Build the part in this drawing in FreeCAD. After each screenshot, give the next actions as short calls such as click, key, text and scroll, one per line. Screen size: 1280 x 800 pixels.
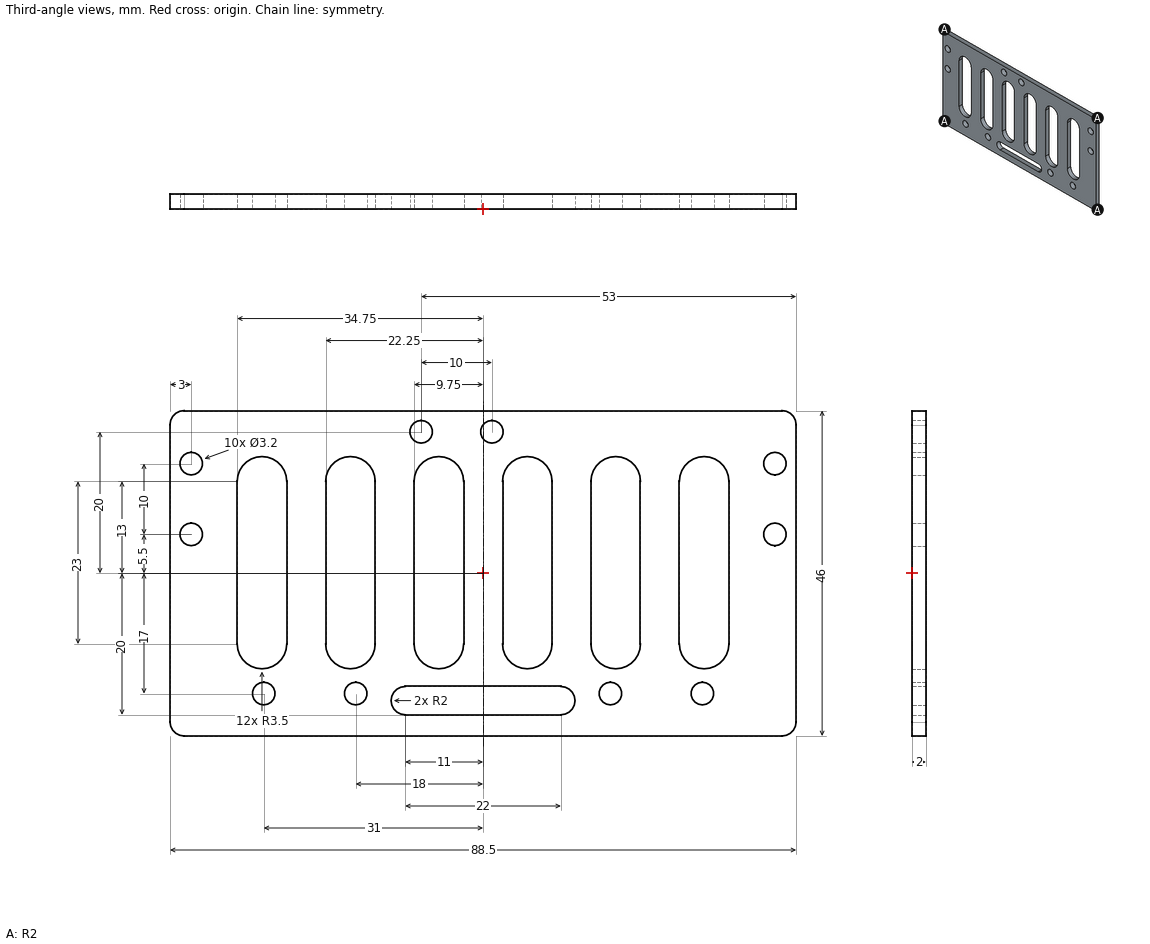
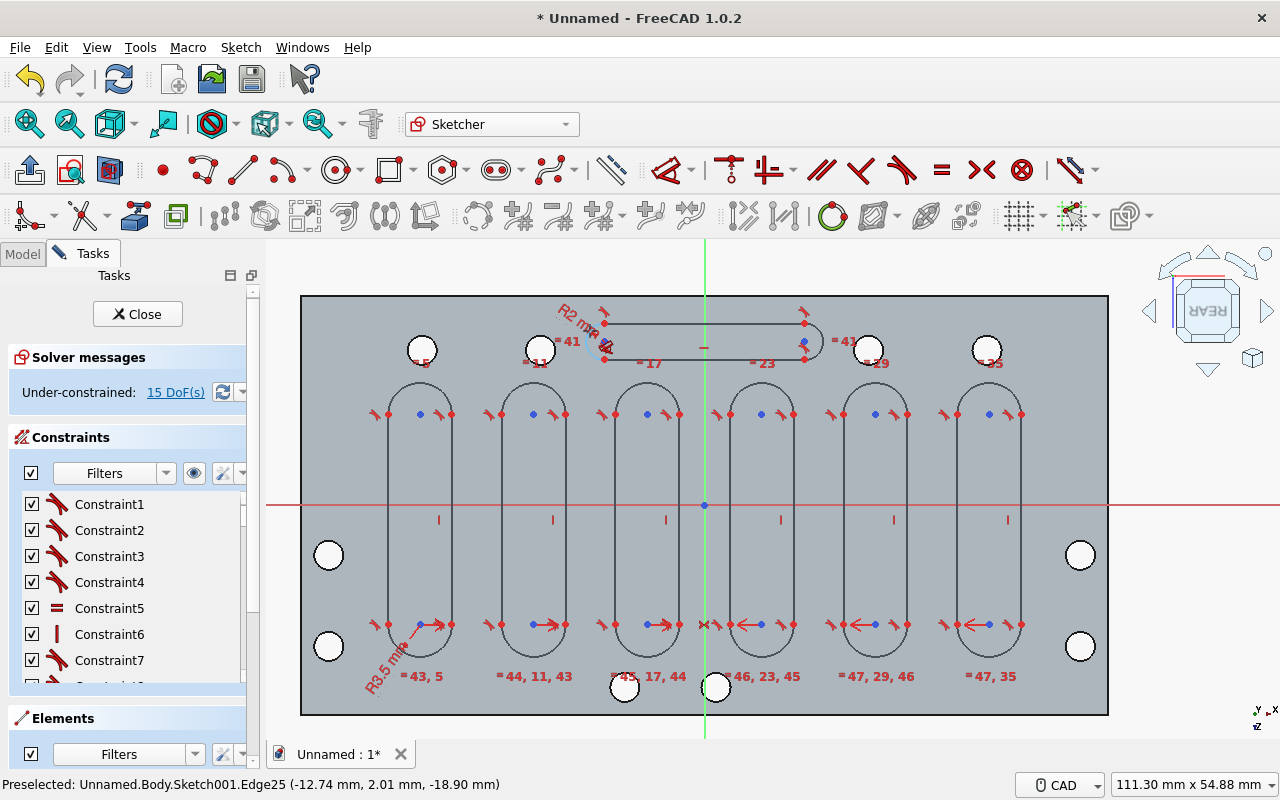
click(388, 562)
click(354, 520)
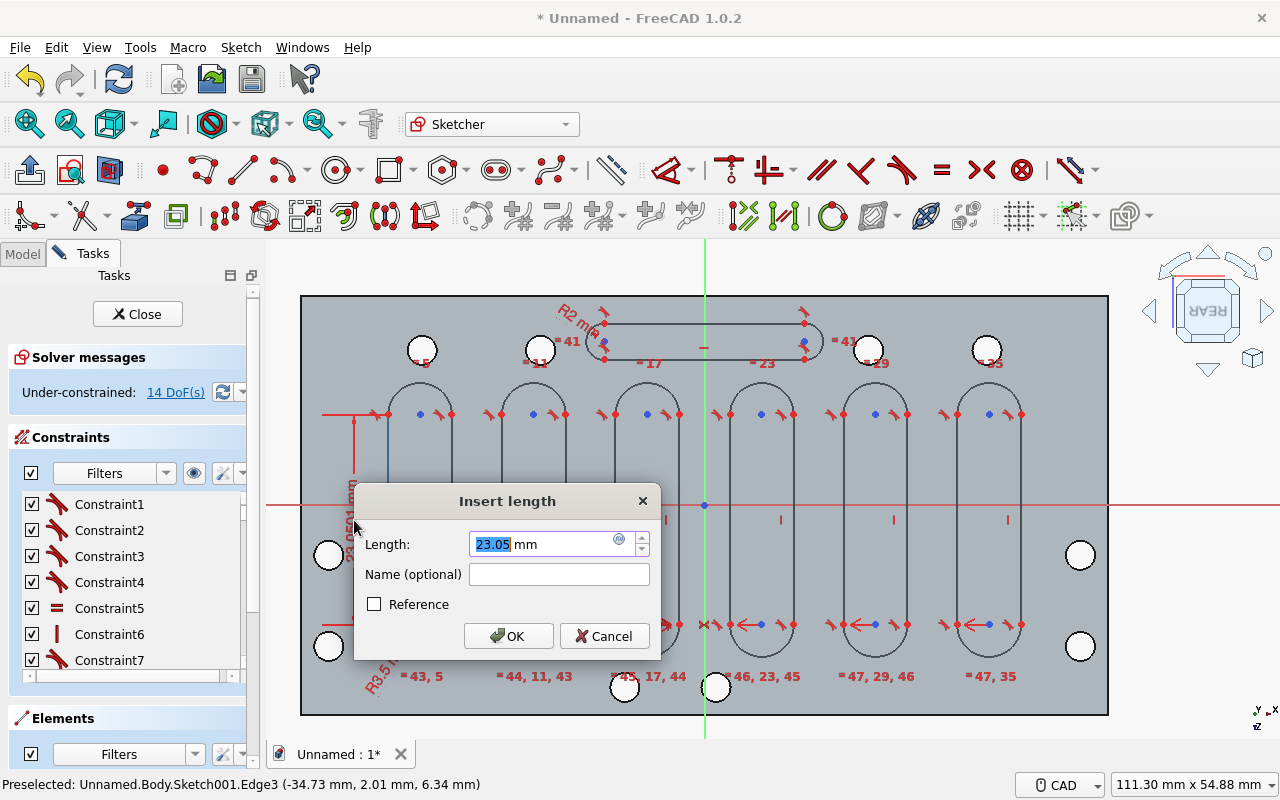
text(23)
key(Return)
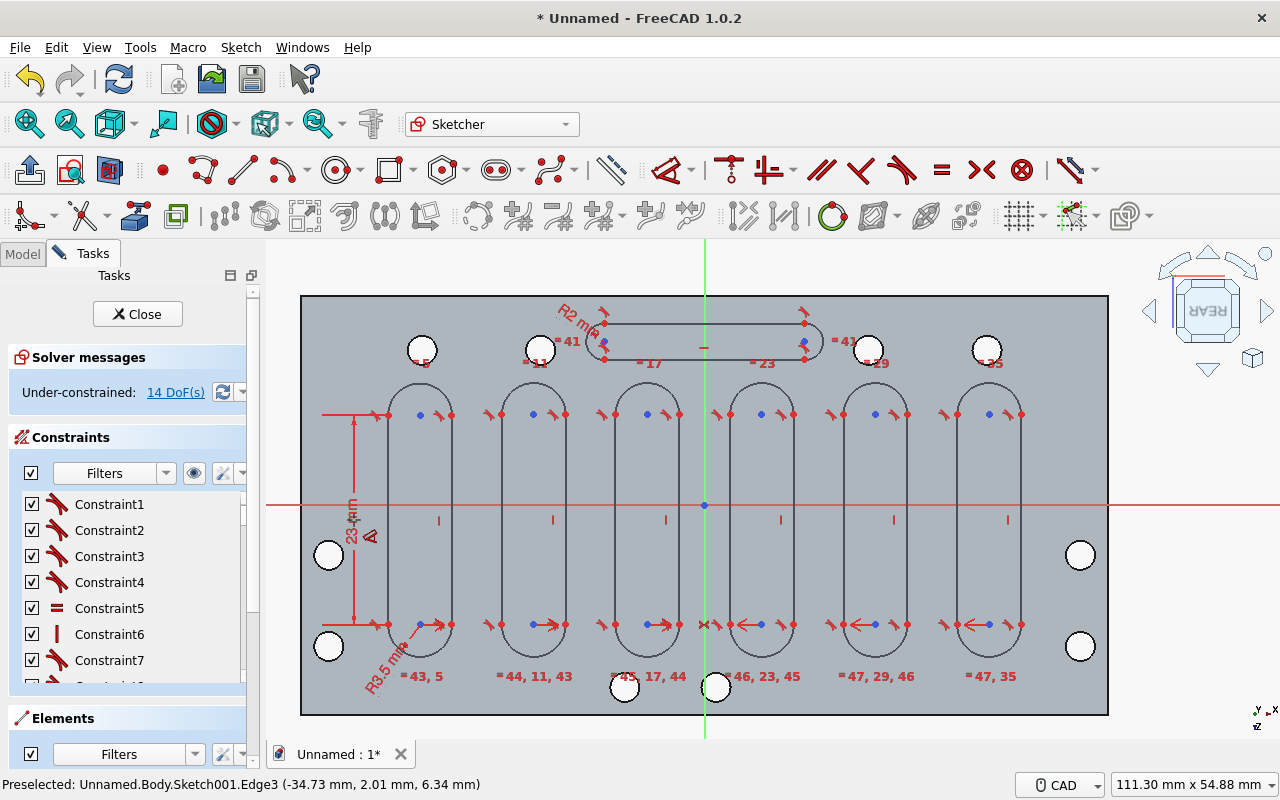
click(502, 562)
click(468, 520)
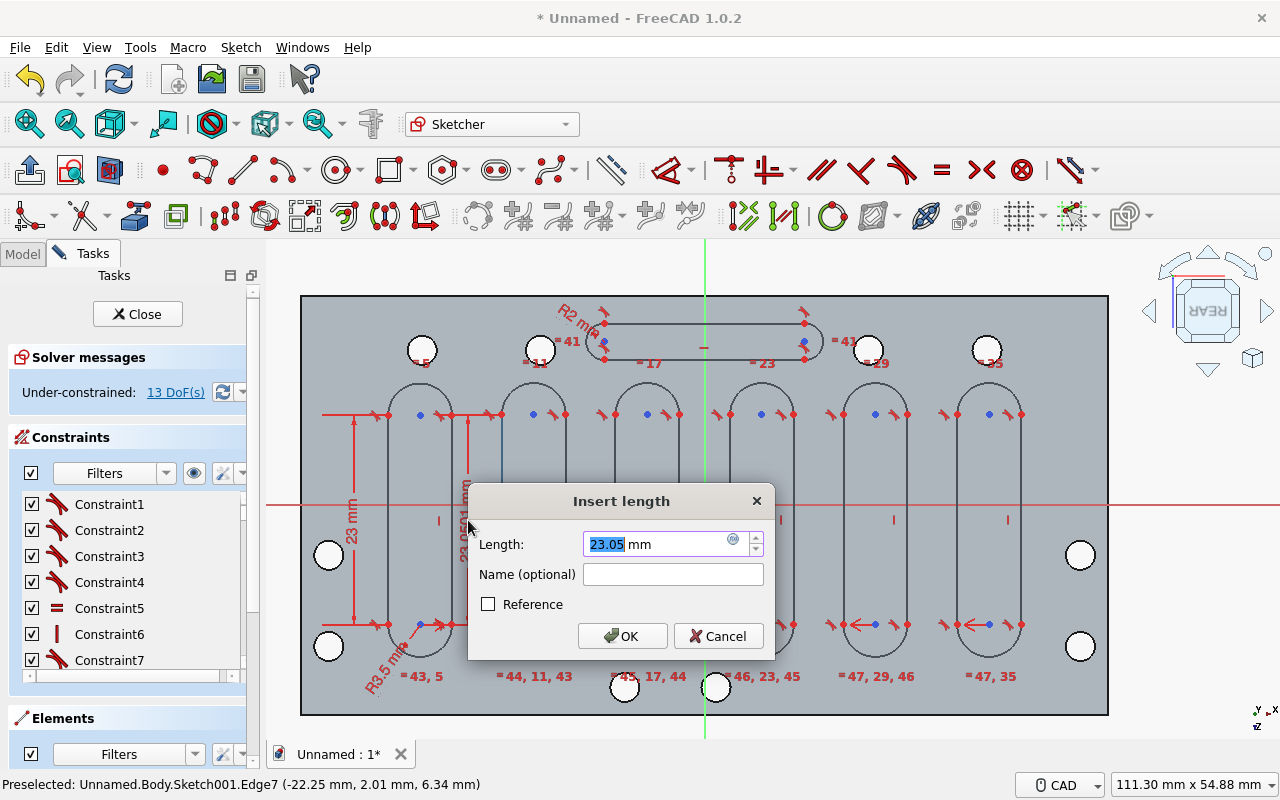
text(23)
key(Return)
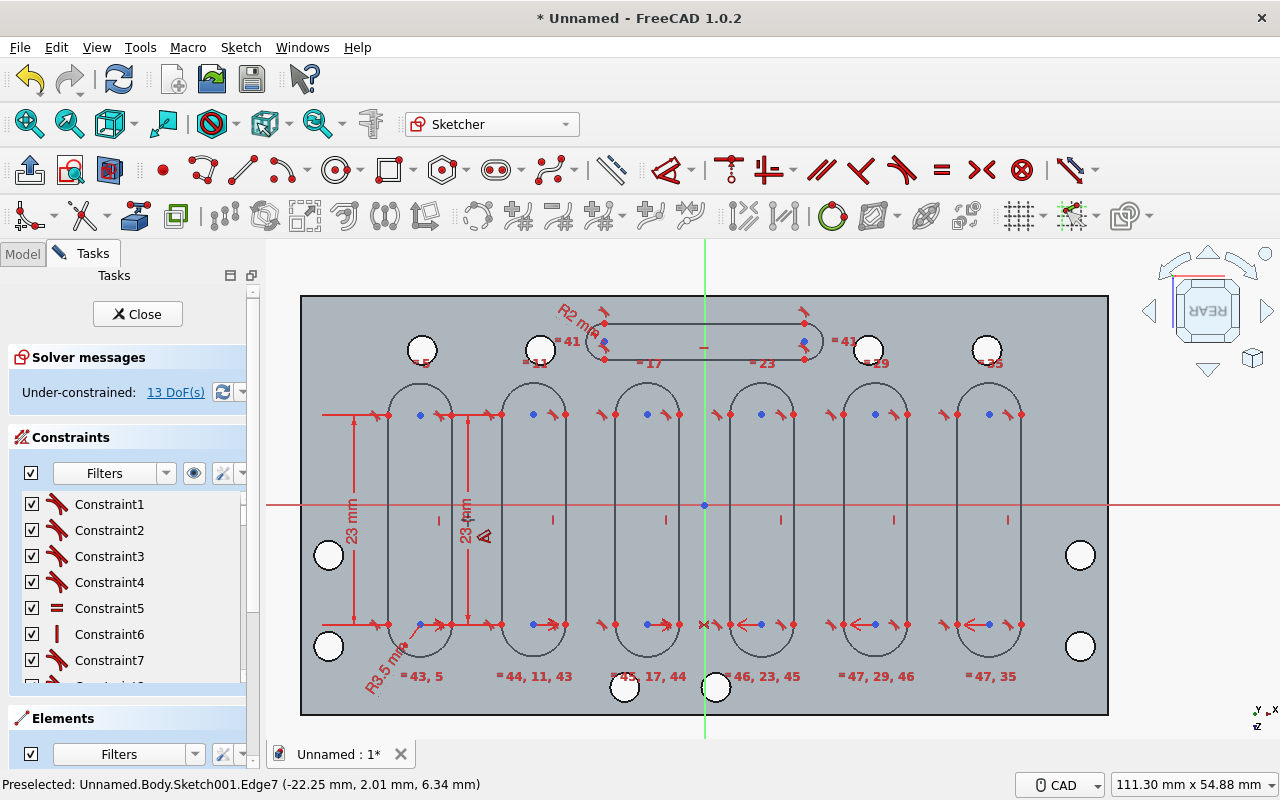
click(615, 562)
click(581, 520)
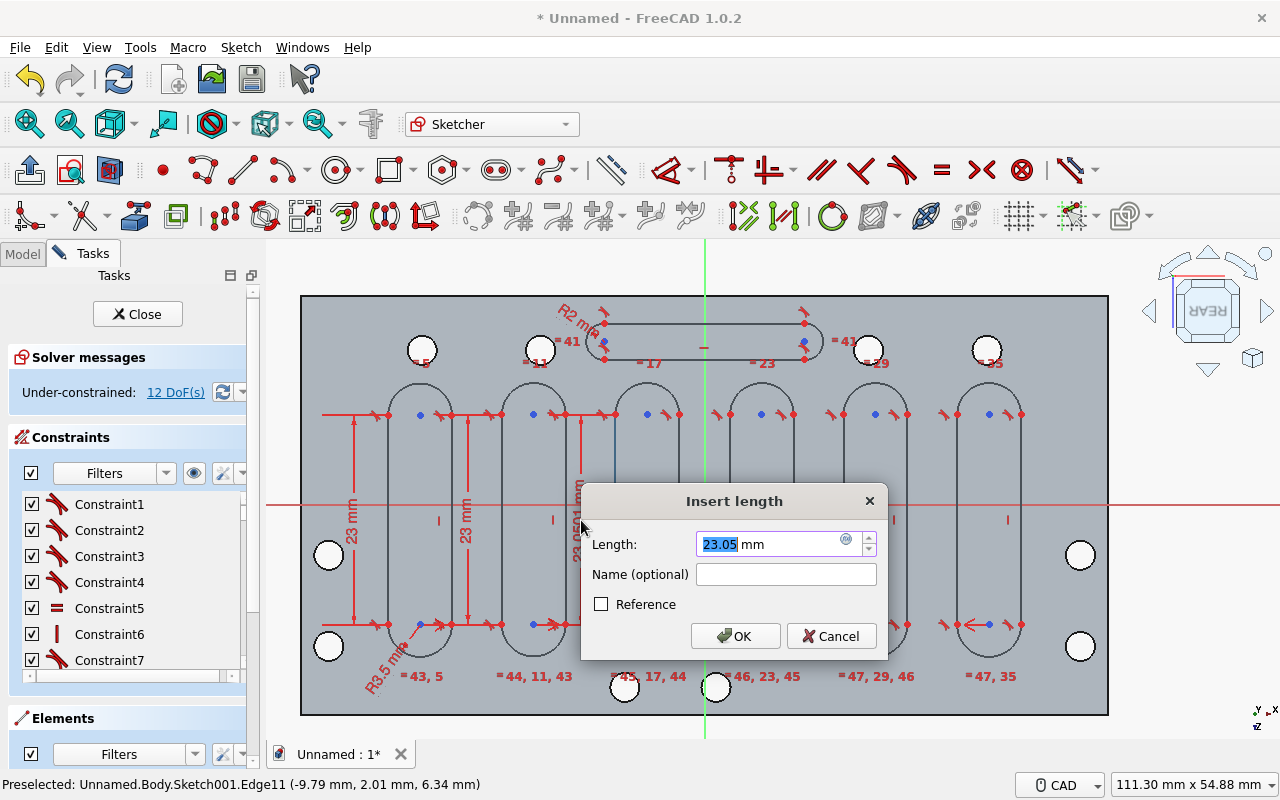
text(23)
key(Return)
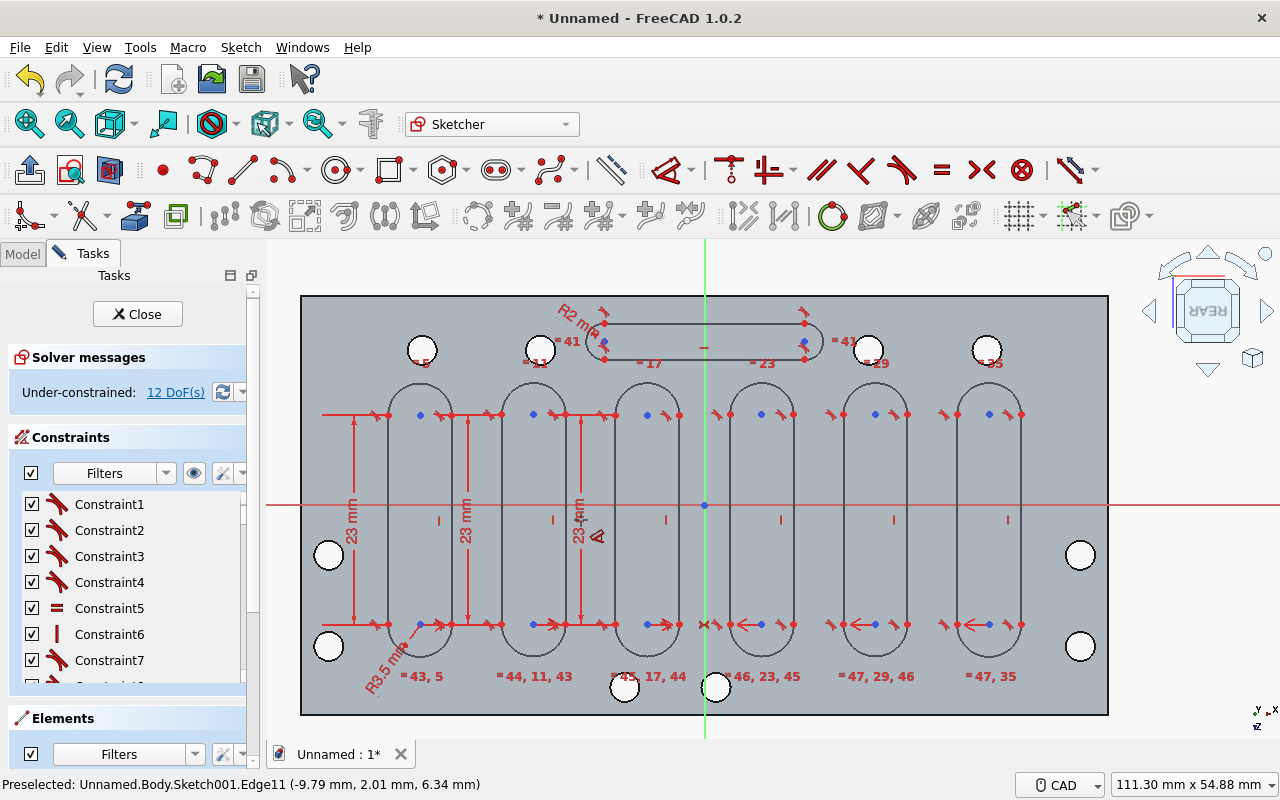
click(730, 562)
click(764, 520)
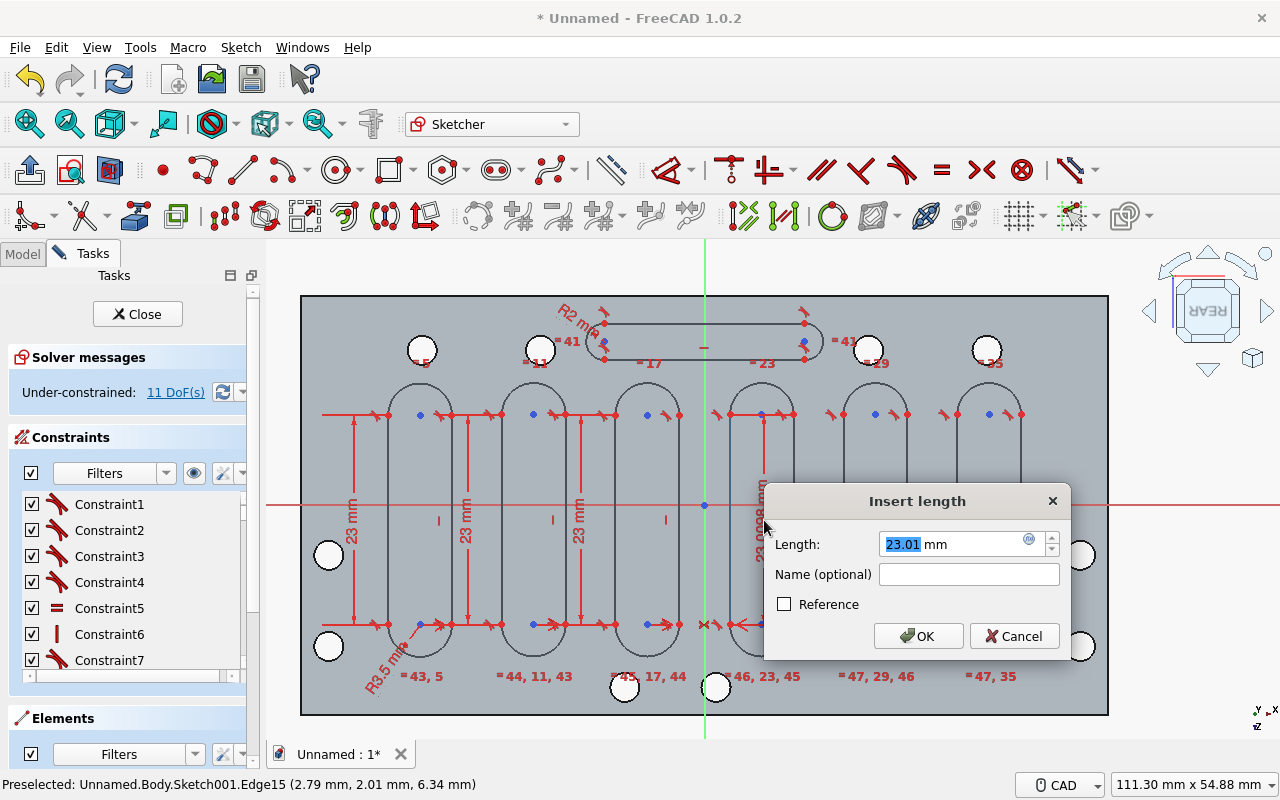
text(23)
key(Return)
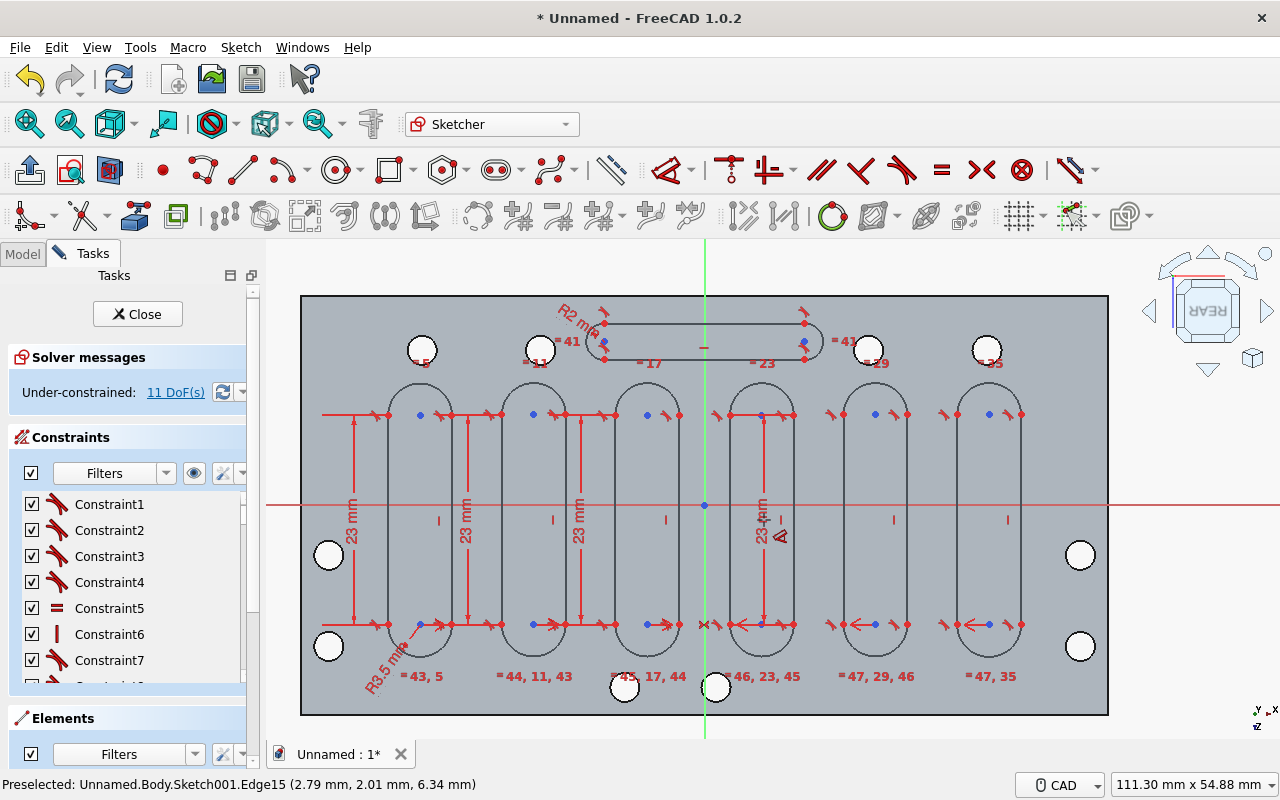
click(844, 562)
click(878, 520)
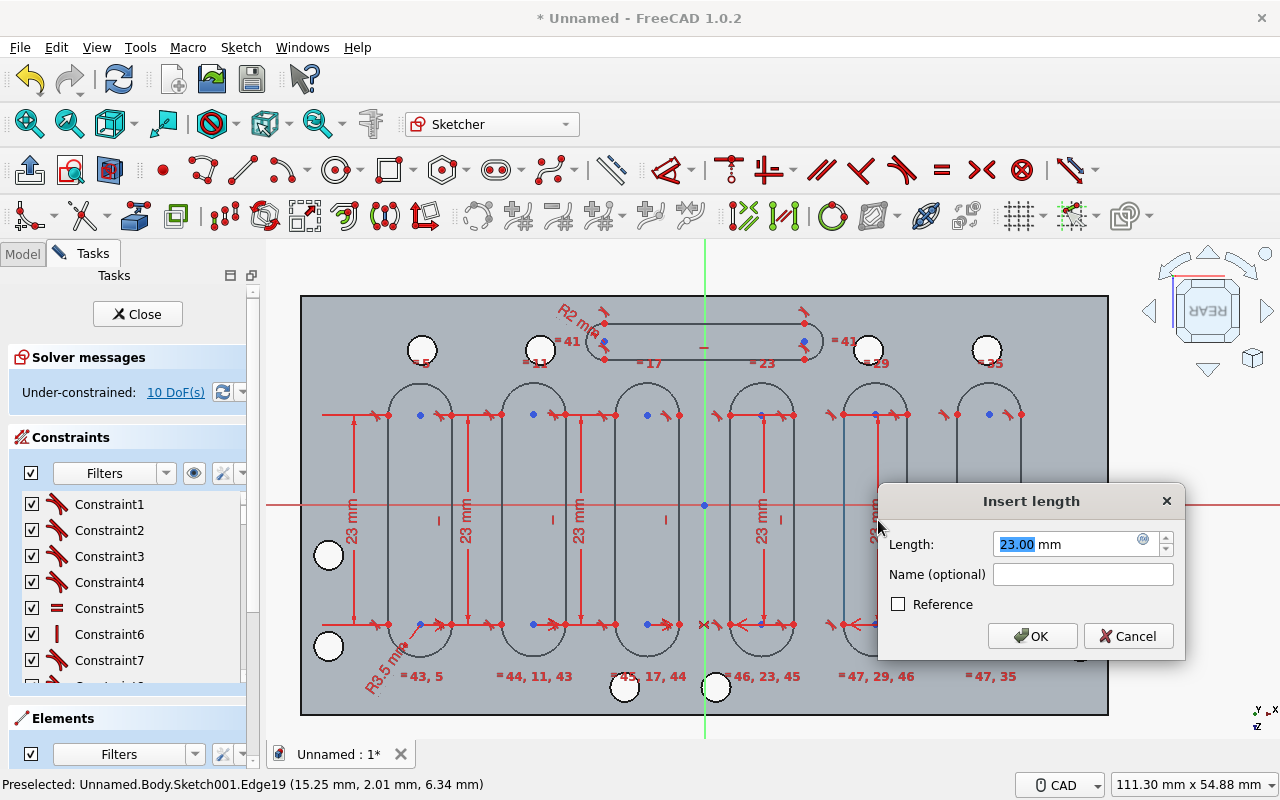
text(23)
key(Return)